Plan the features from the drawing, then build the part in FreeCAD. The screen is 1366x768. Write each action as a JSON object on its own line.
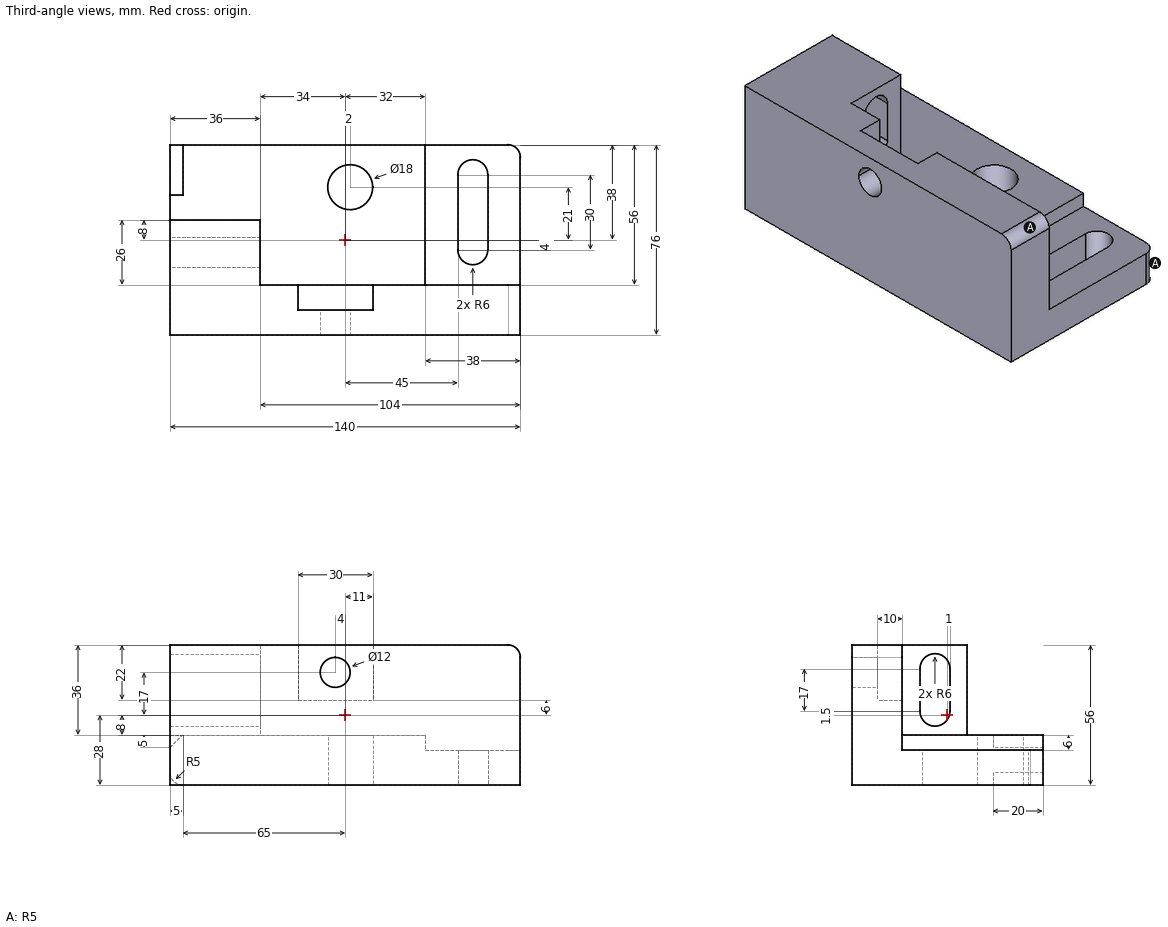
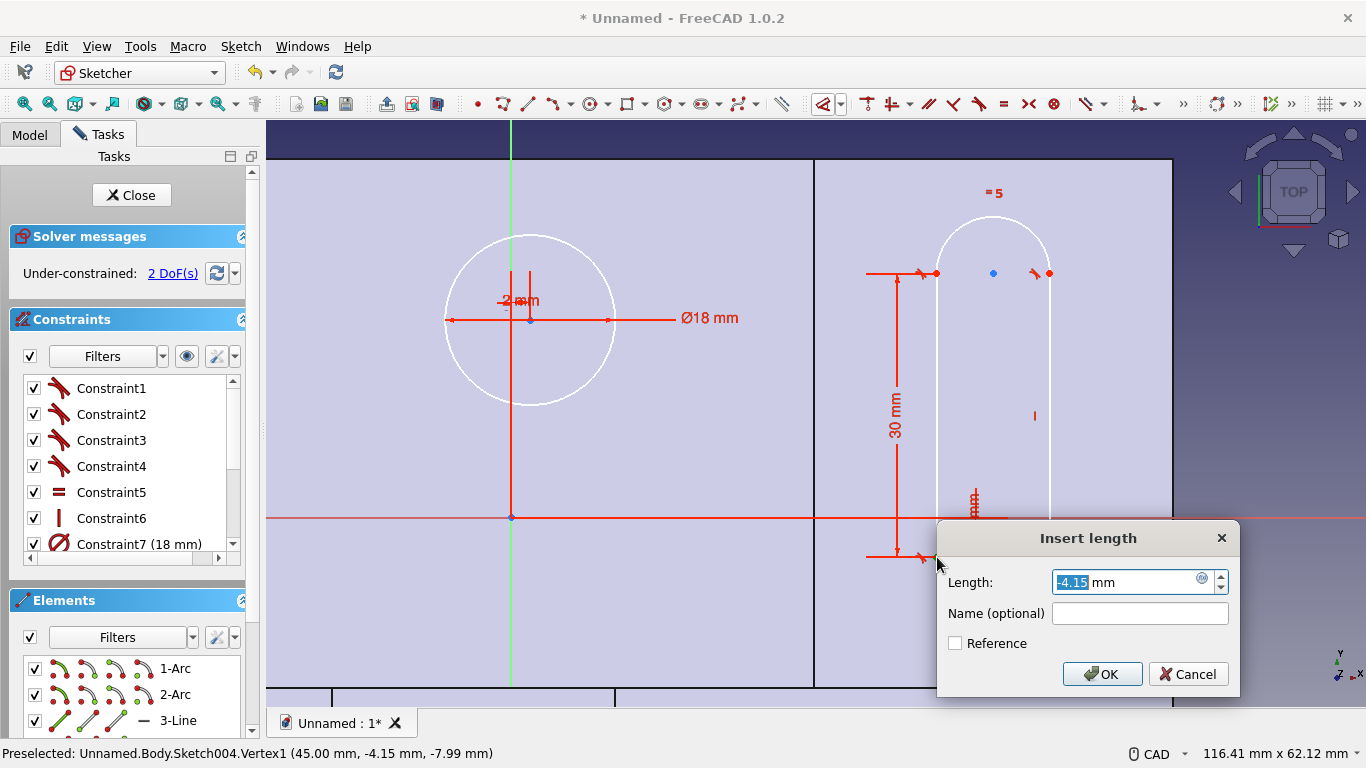
{"action": "type", "text": "-4"}
{"action": "key", "text": "Return"}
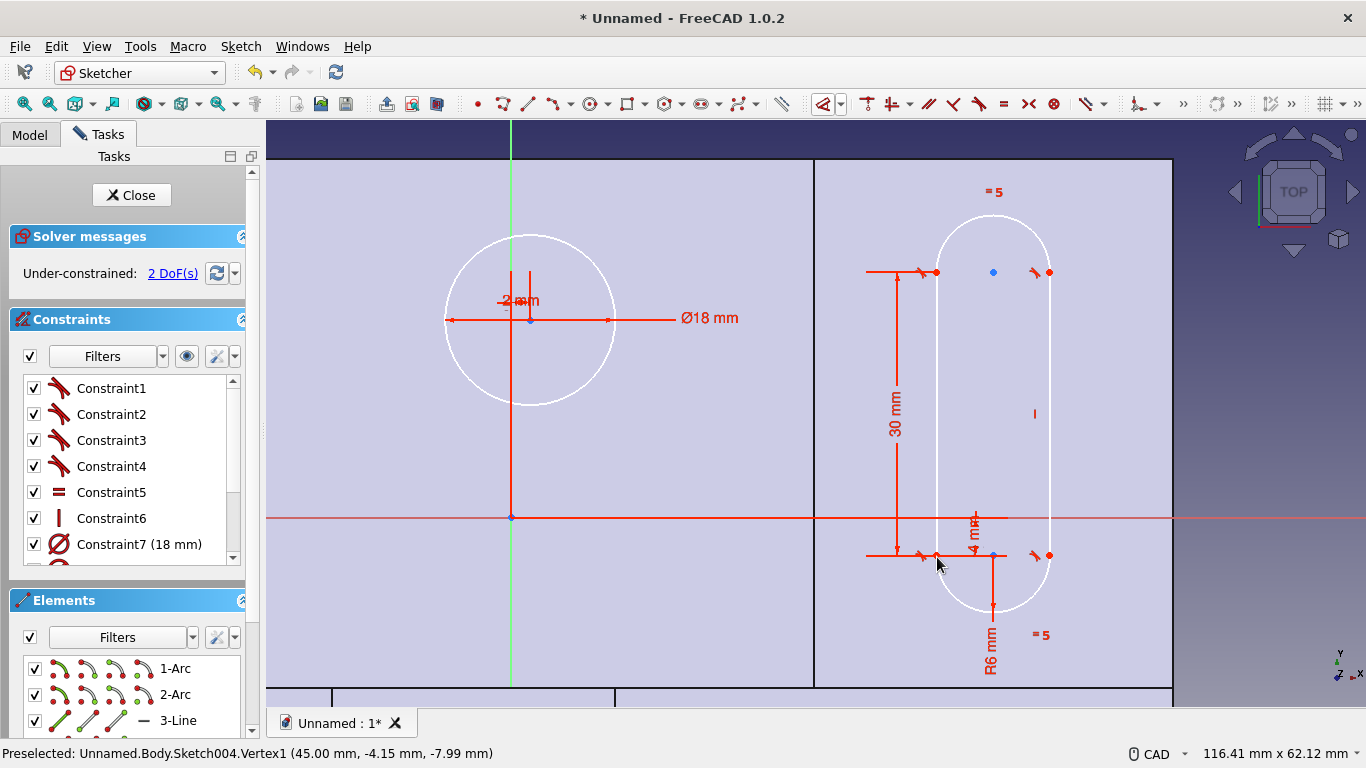
{"action": "left_click", "coordinate": [530, 320]}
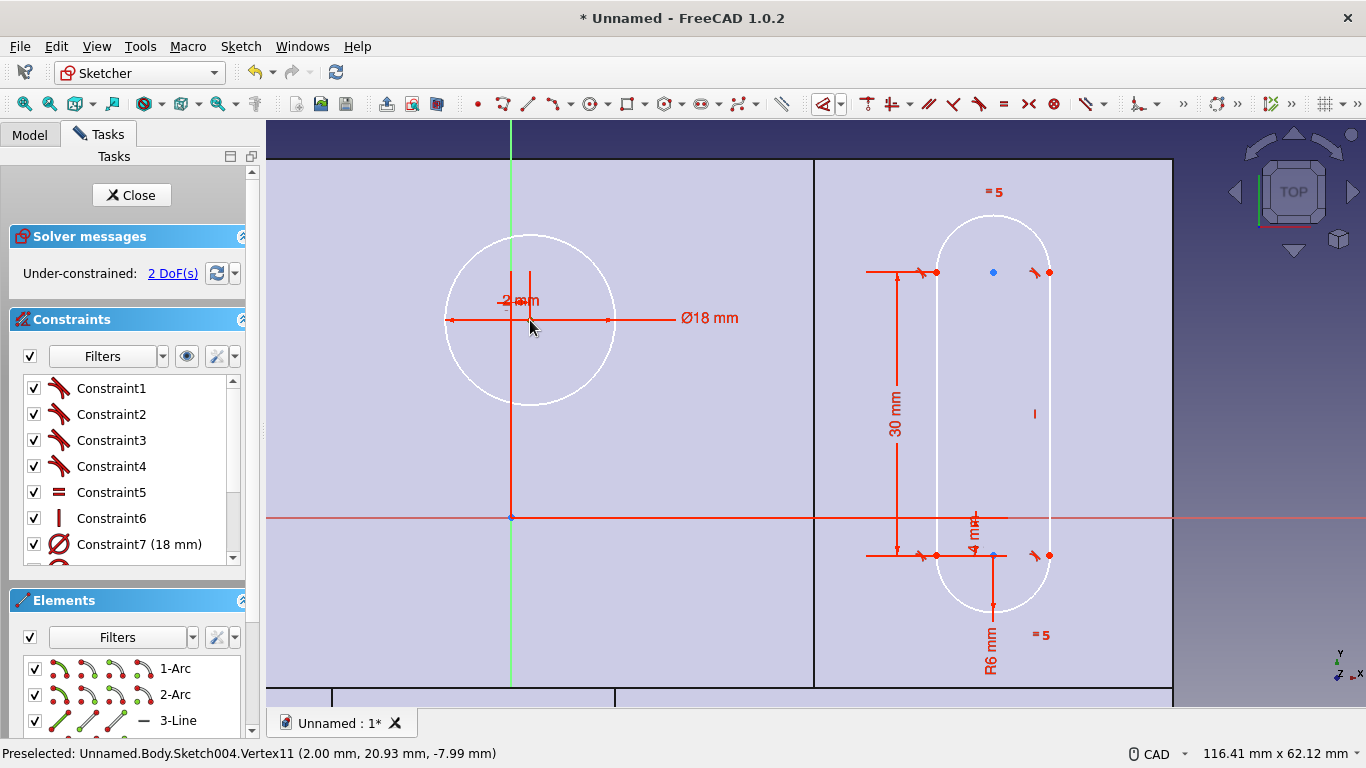
{"action": "key", "text": "i"}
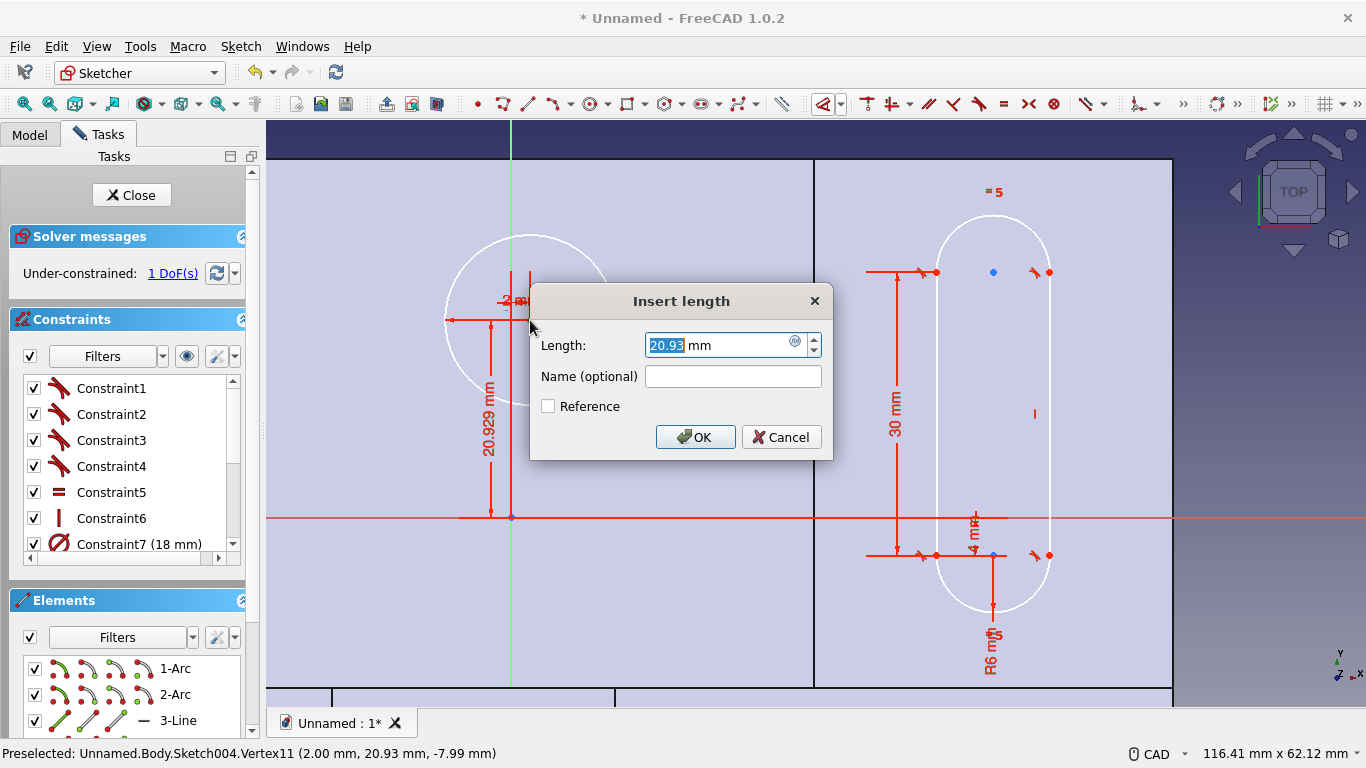
{"action": "type", "text": "21"}
{"action": "key", "text": "Return"}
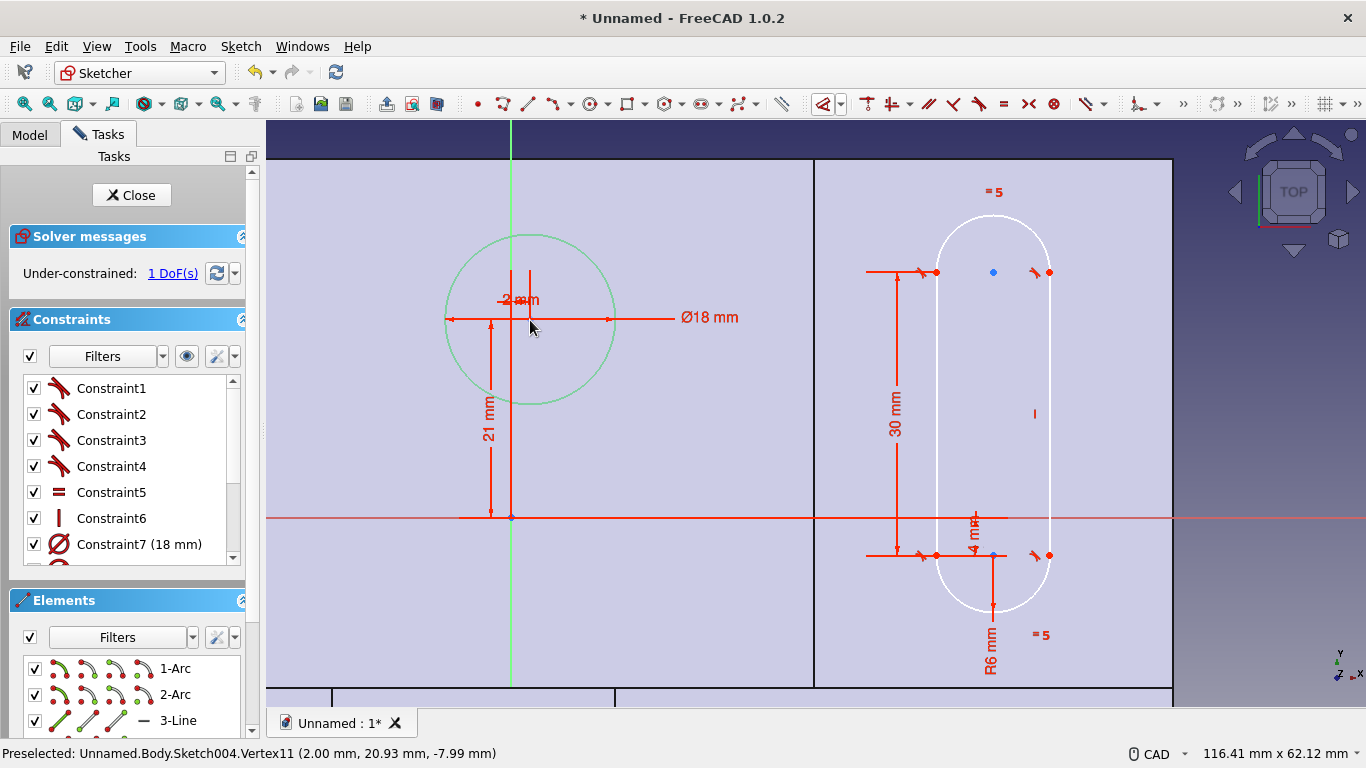
{"action": "left_click", "coordinate": [937, 556]}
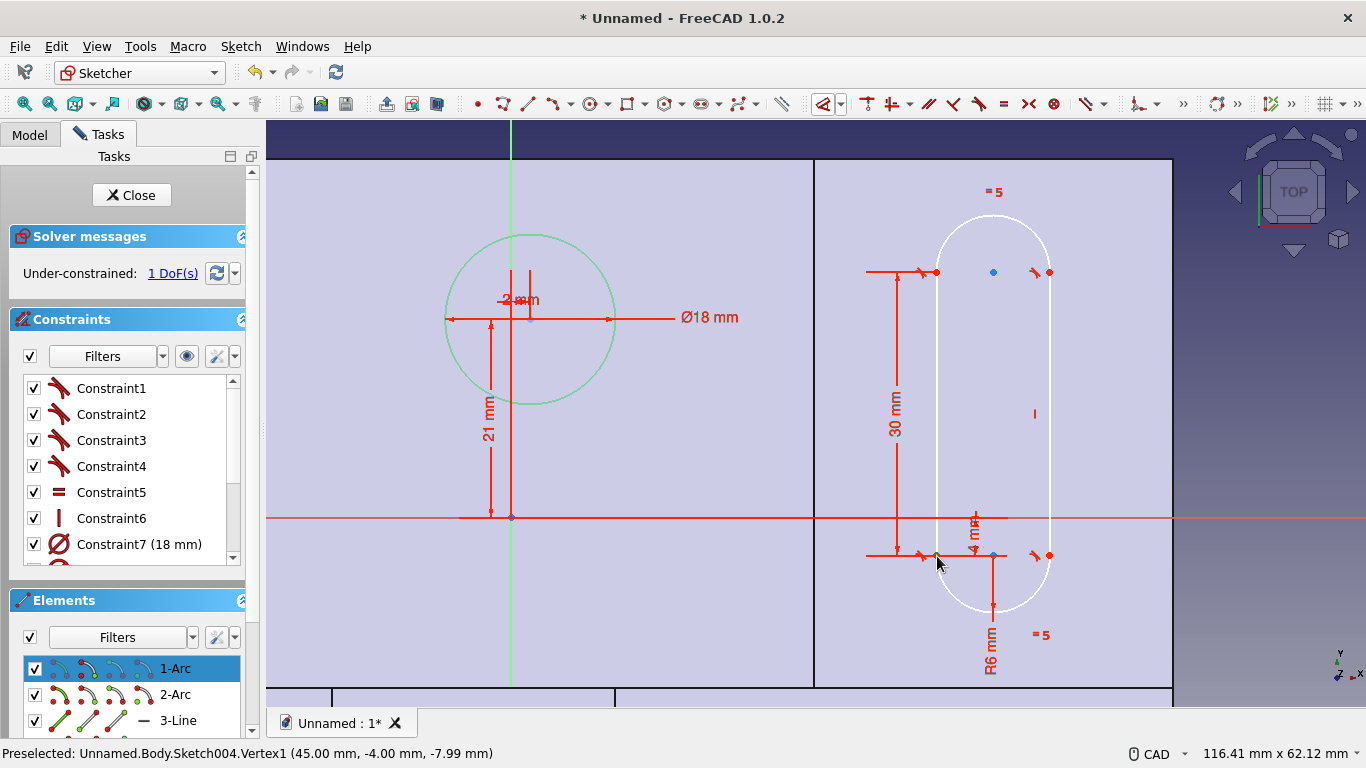
{"action": "left_click", "coordinate": [840, 104]}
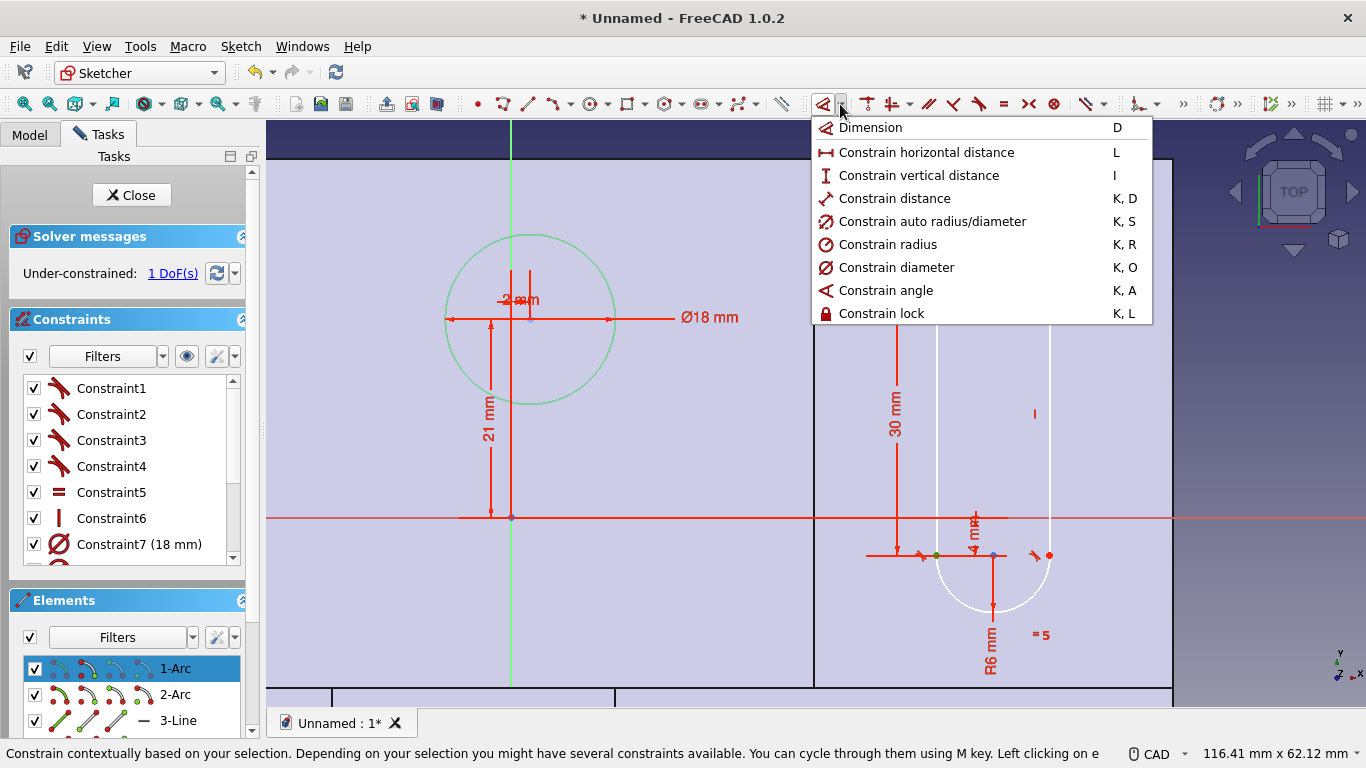
{"action": "left_click", "coordinate": [982, 152]}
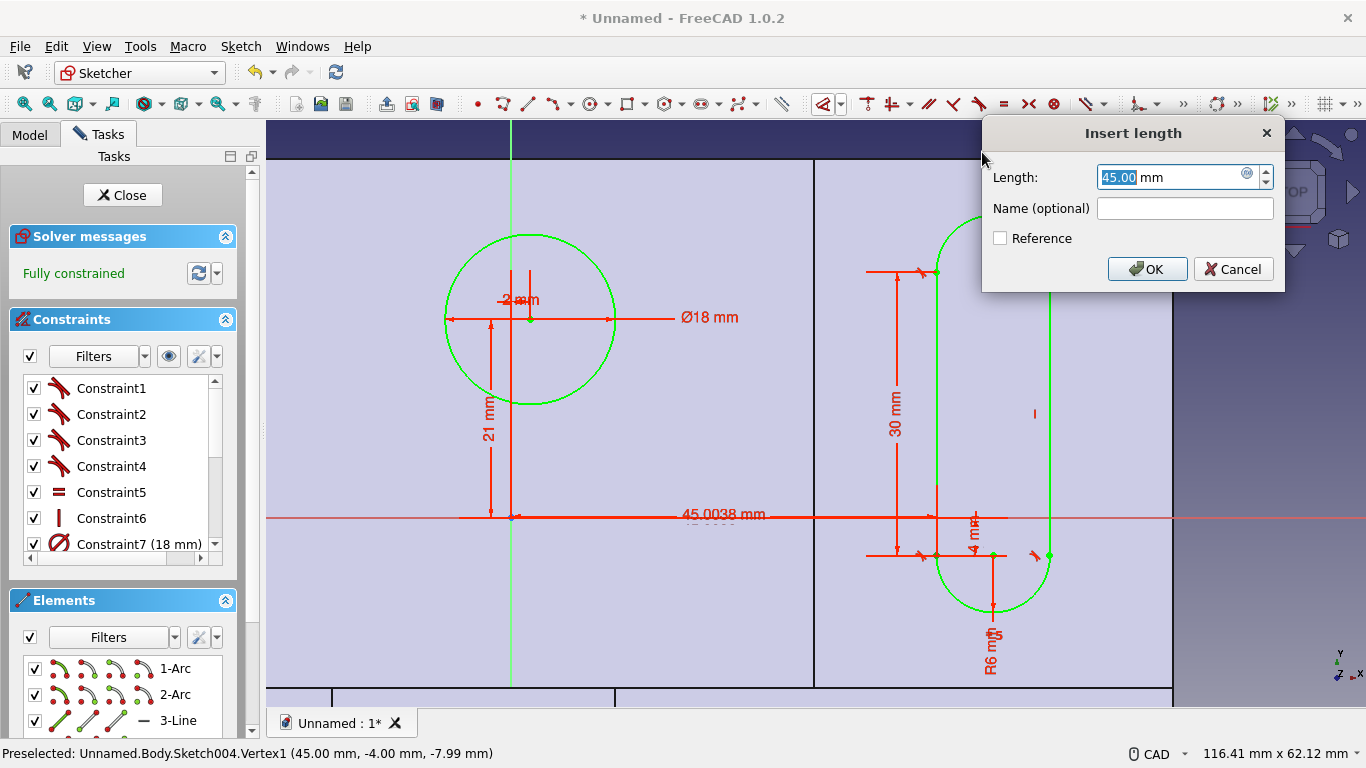
{"action": "type", "text": "45"}
{"action": "key", "text": "Return"}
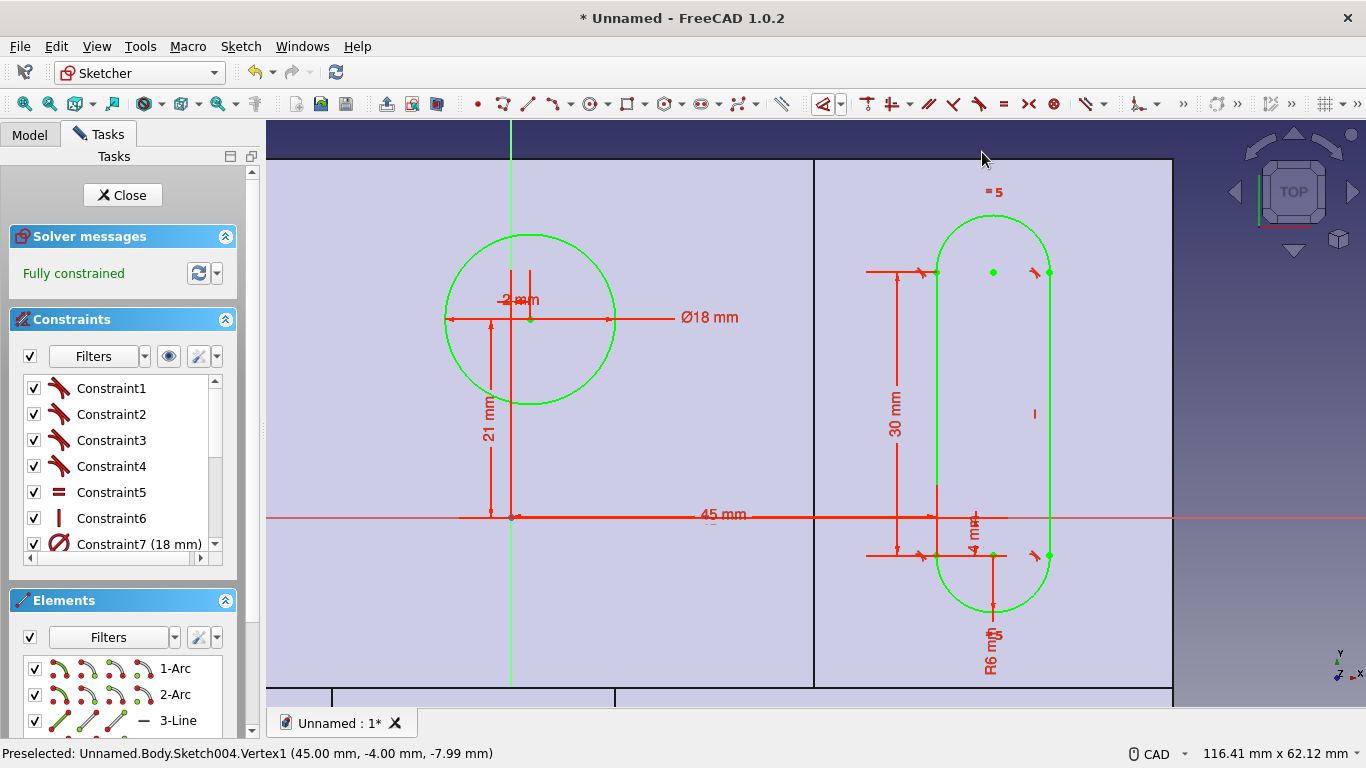
{"action": "left_click", "coordinate": [123, 195]}